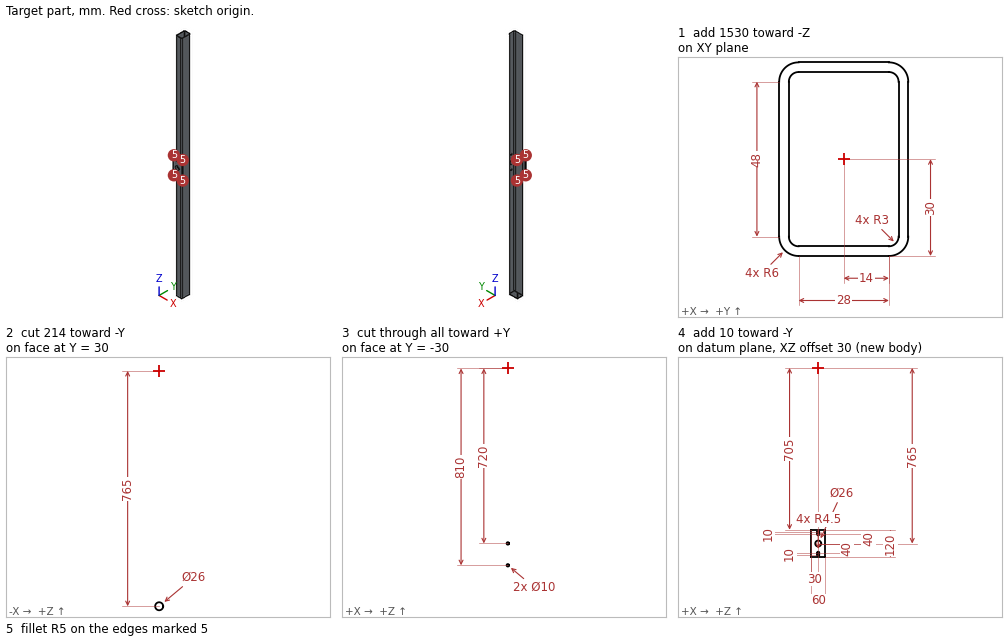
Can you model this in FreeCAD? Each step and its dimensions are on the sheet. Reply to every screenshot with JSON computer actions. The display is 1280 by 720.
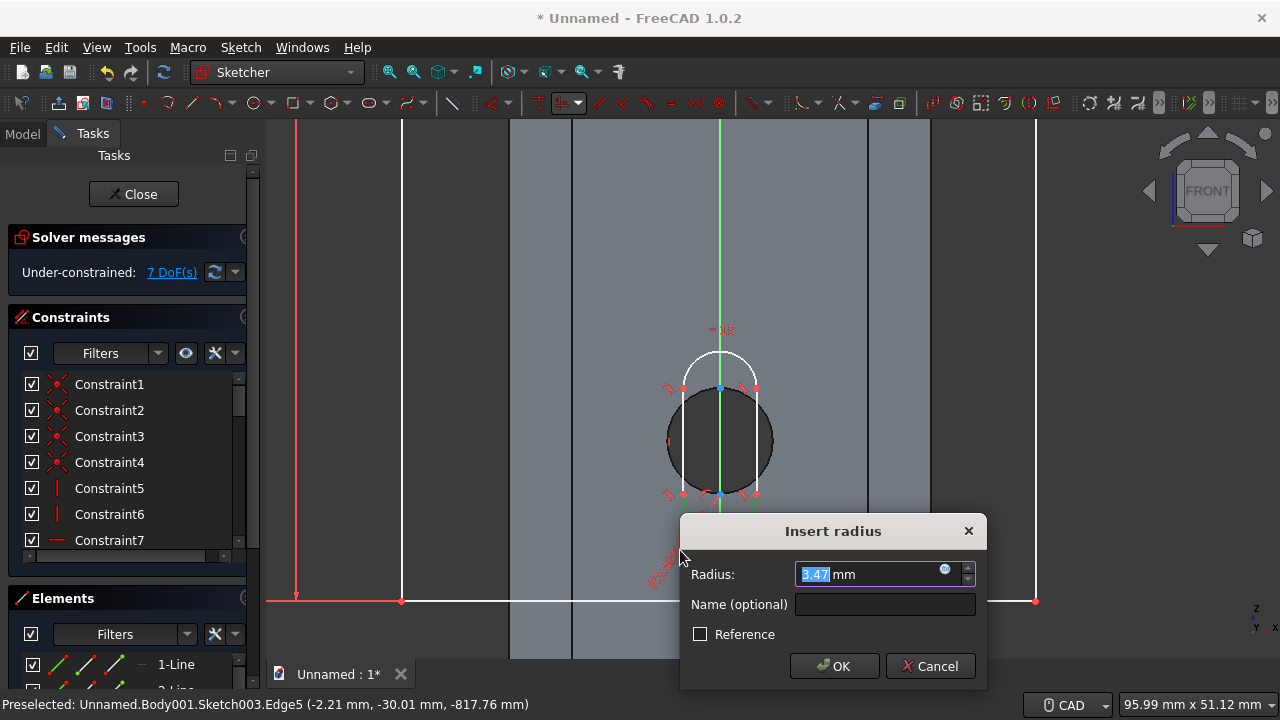
{"action": "type", "text": "4.5"}
{"action": "key", "text": "Return"}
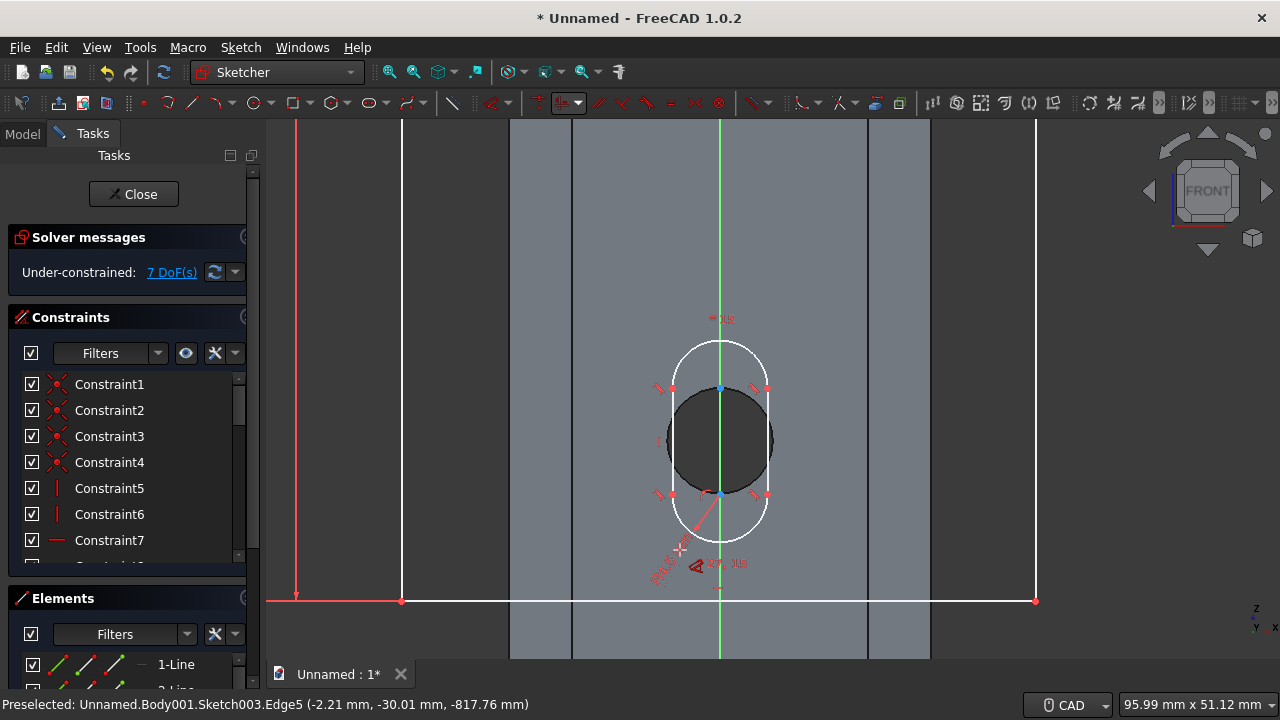
{"action": "left_click", "coordinate": [673, 463]}
{"action": "left_click", "coordinate": [639, 441]}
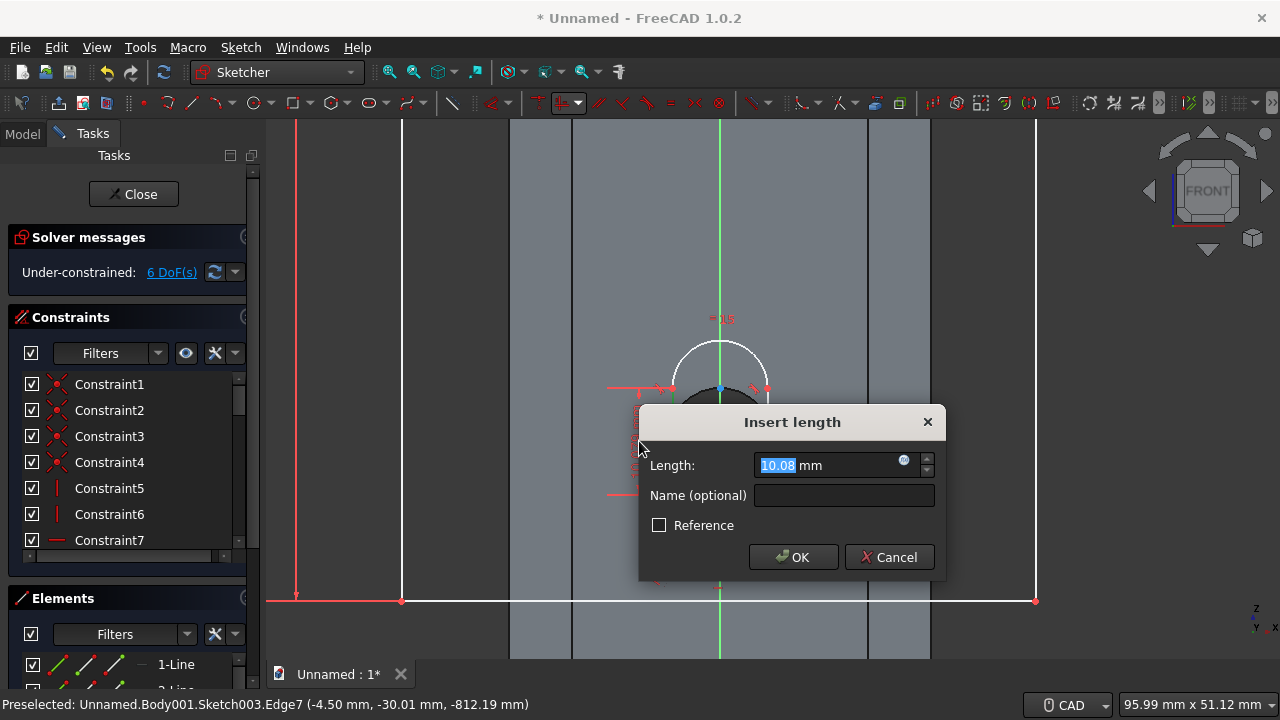
{"action": "type", "text": "10"}
{"action": "key", "text": "Return"}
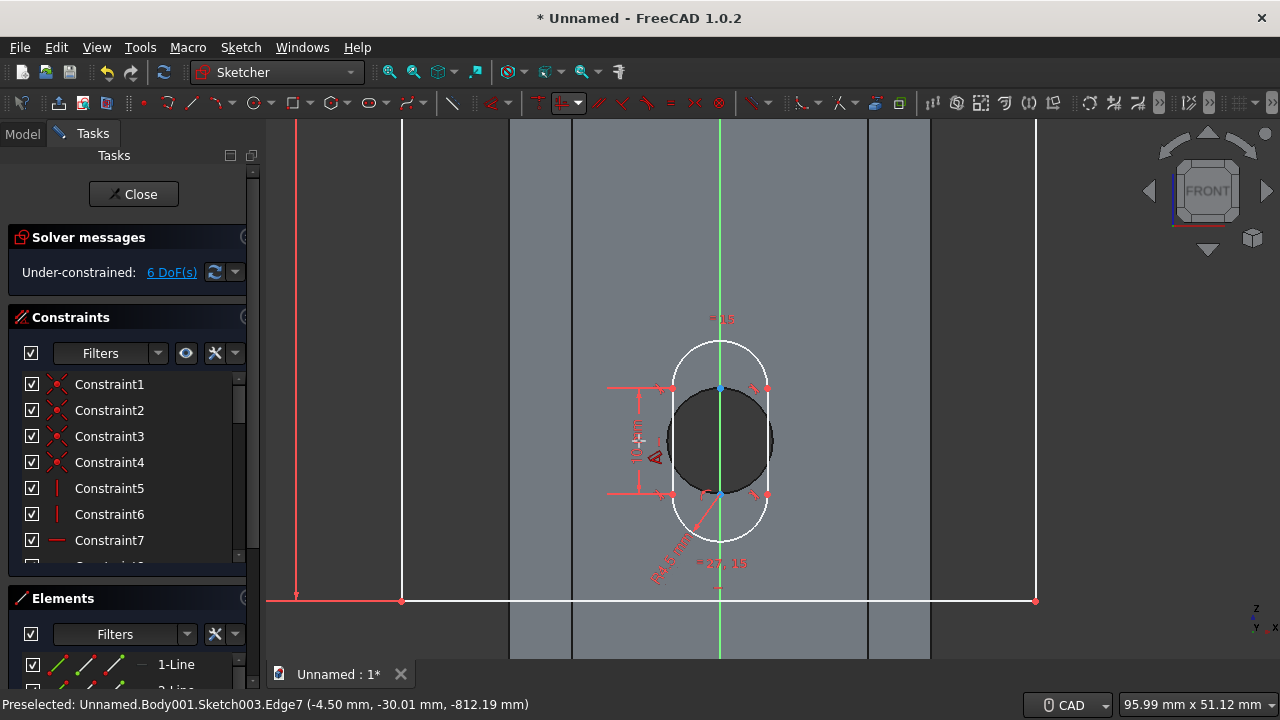
{"action": "scroll", "coordinate": [699, 528], "scroll_direction": "down", "scroll_amount": 7}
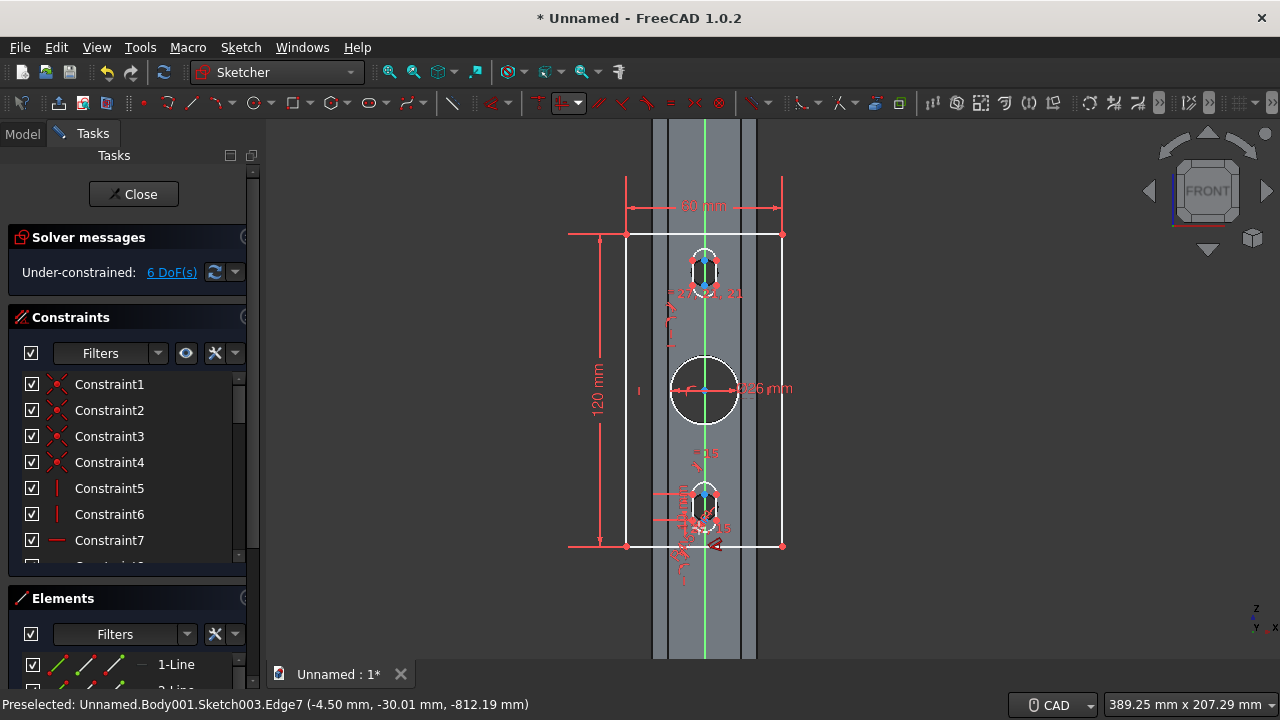
{"action": "scroll", "coordinate": [693, 278], "scroll_direction": "up", "scroll_amount": 4}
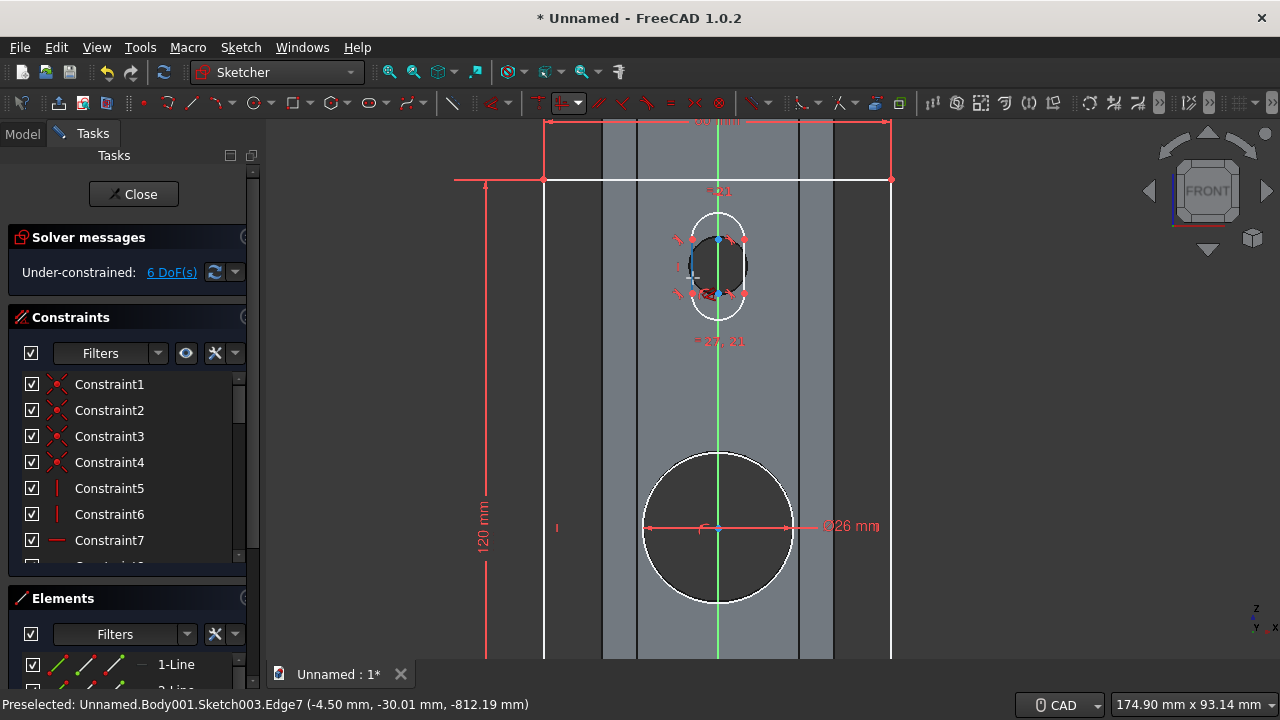
{"action": "left_click", "coordinate": [692, 277]}
{"action": "left_click", "coordinate": [658, 266]}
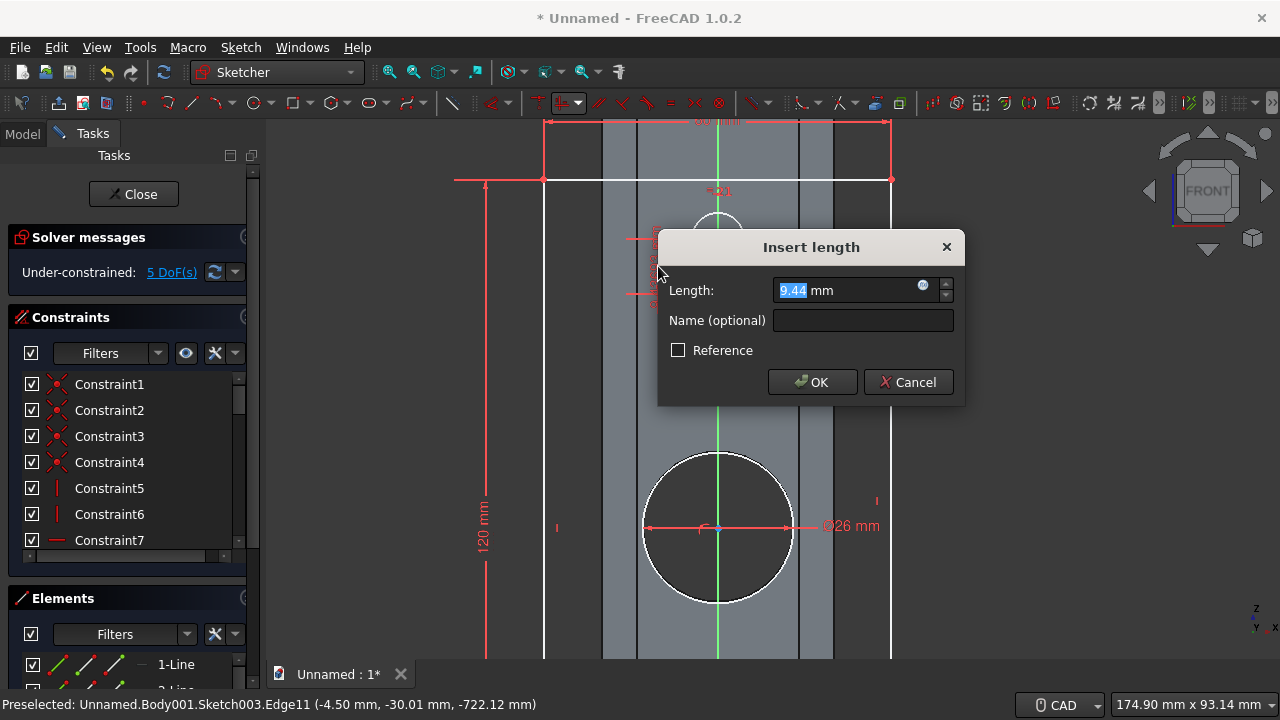
{"action": "type", "text": "10"}
{"action": "key", "text": "Return"}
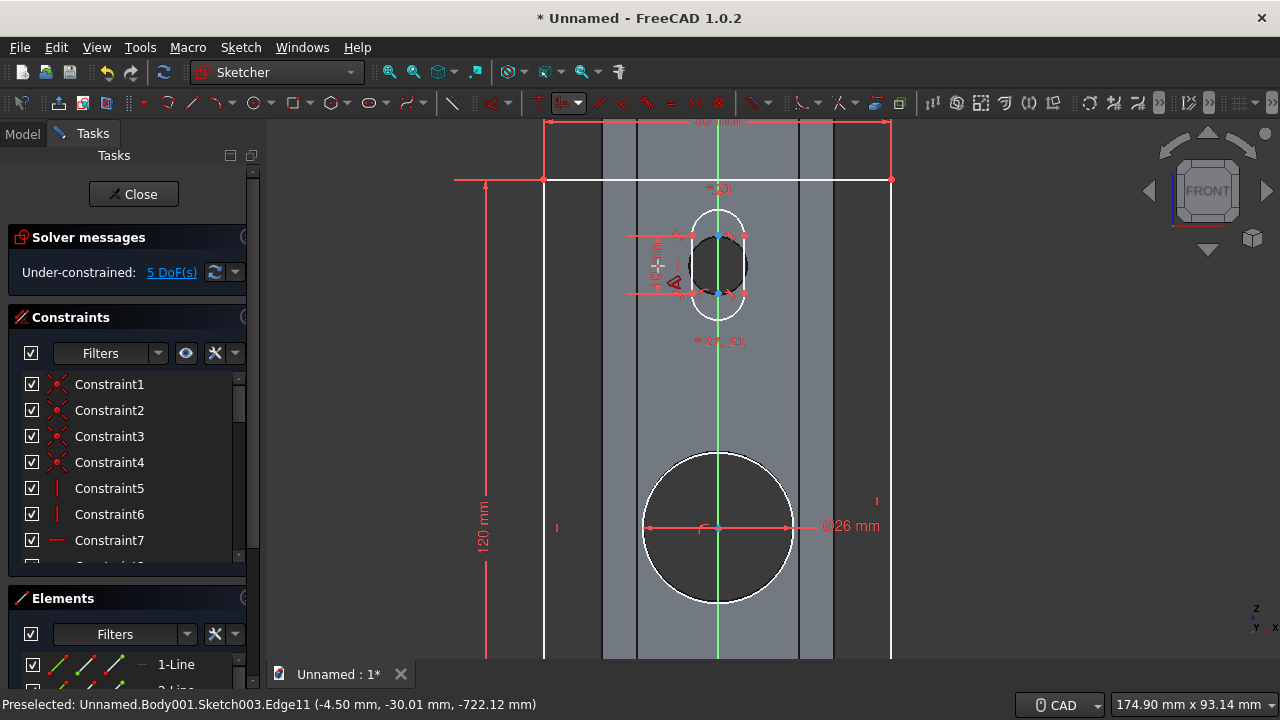
{"action": "left_click", "coordinate": [544, 180]}
{"action": "left_click", "coordinate": [631, 214]}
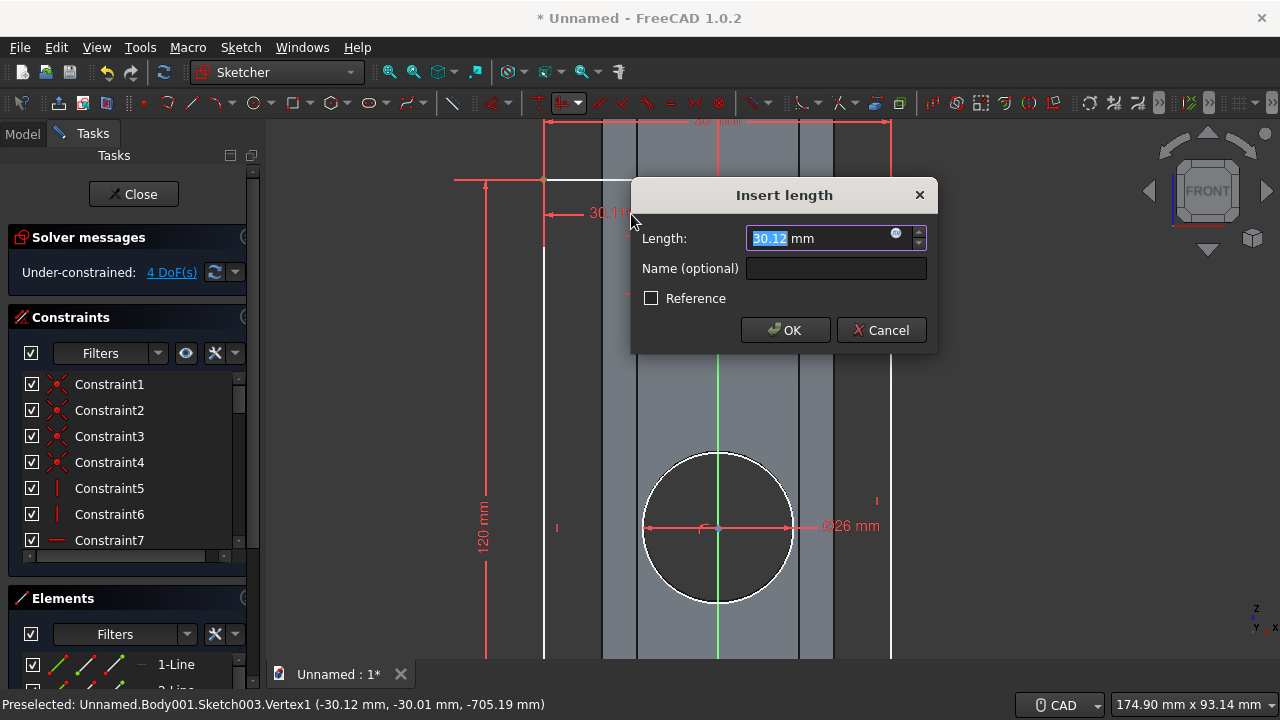
{"action": "type", "text": "30"}
{"action": "key", "text": "Return"}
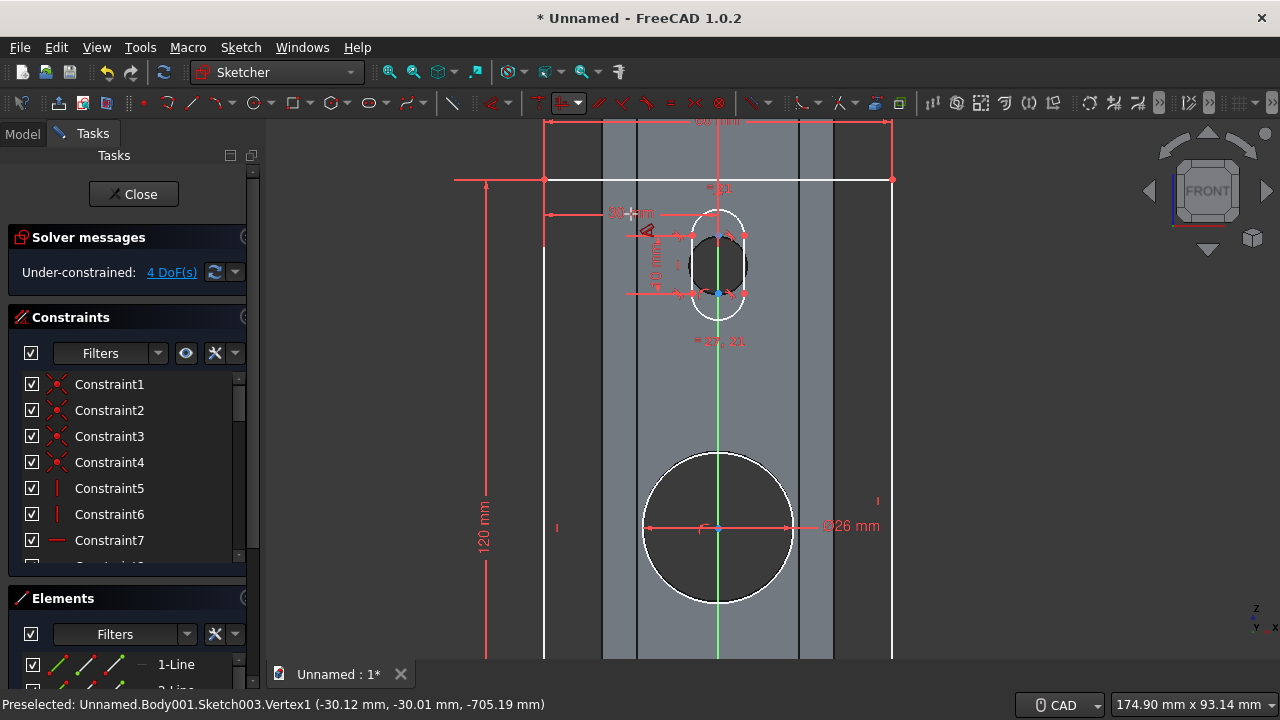
{"action": "left_click", "coordinate": [718, 528]}
{"action": "left_click", "coordinate": [752, 338]}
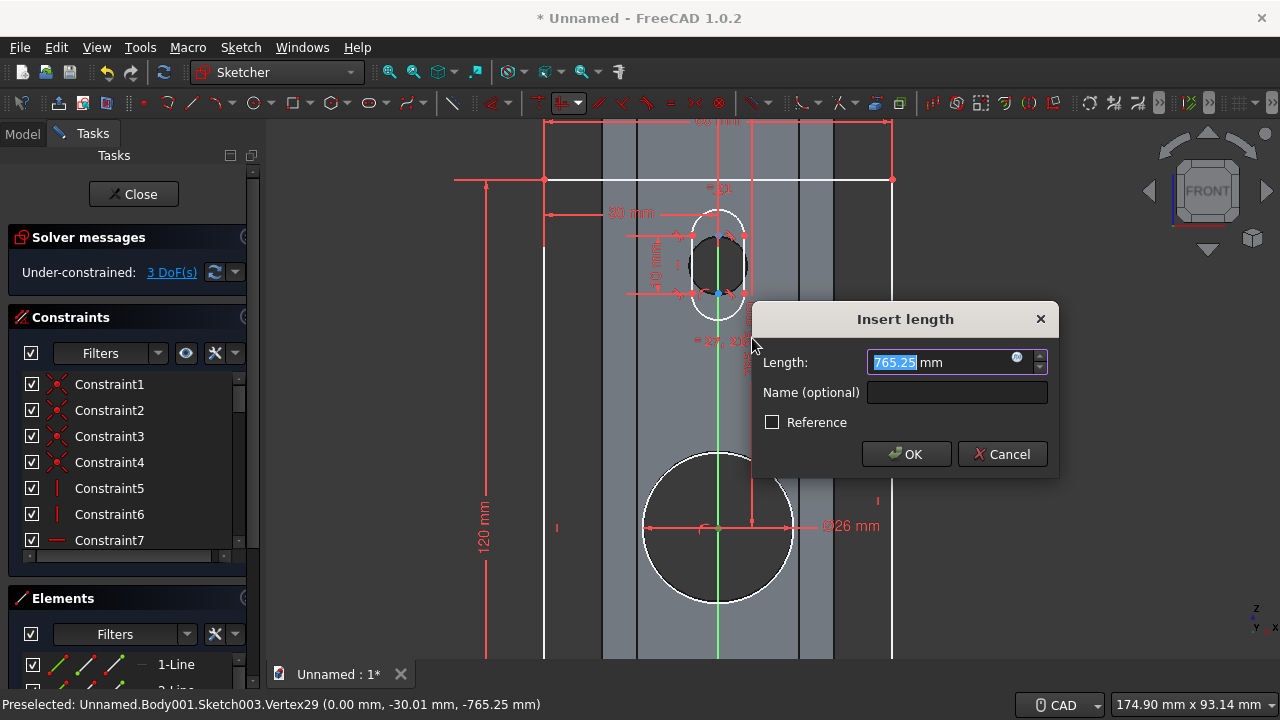
{"action": "type", "text": "765"}
{"action": "key", "text": "Return"}